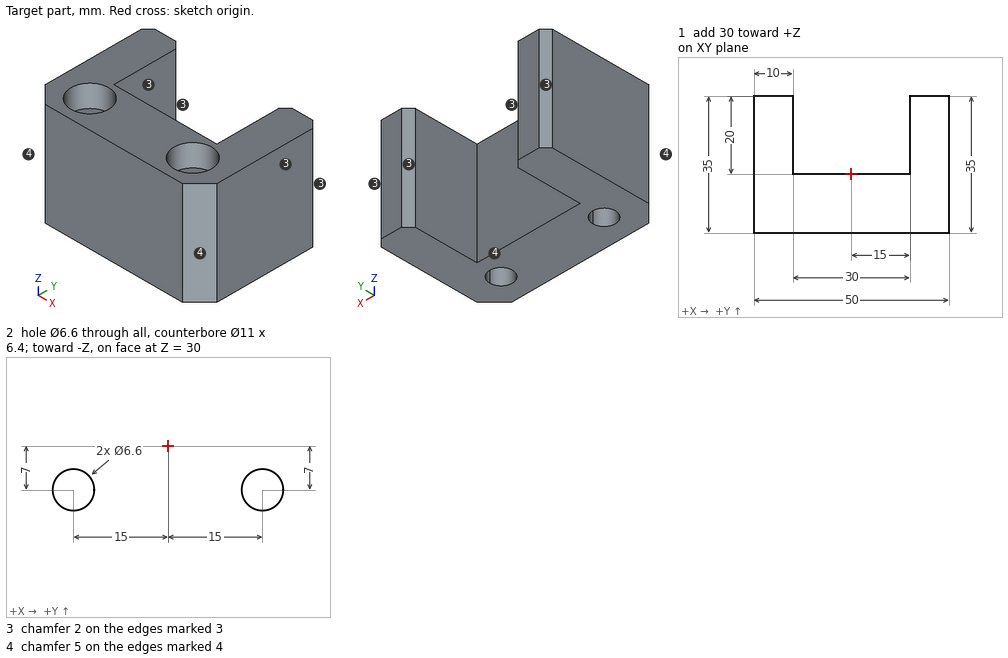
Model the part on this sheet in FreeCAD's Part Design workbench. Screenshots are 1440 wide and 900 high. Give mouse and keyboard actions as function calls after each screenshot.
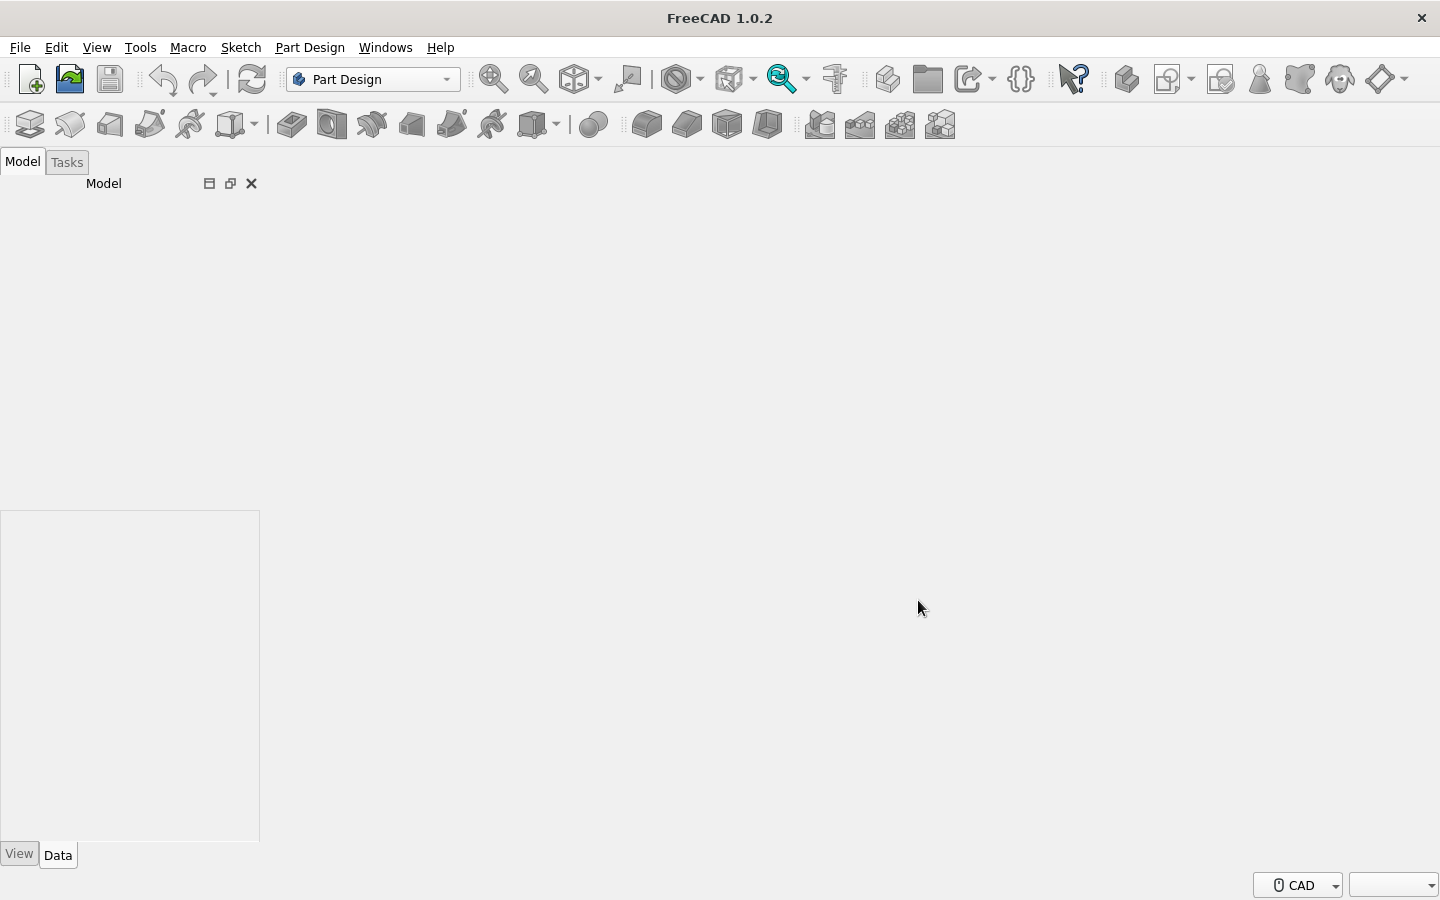
click(30, 80)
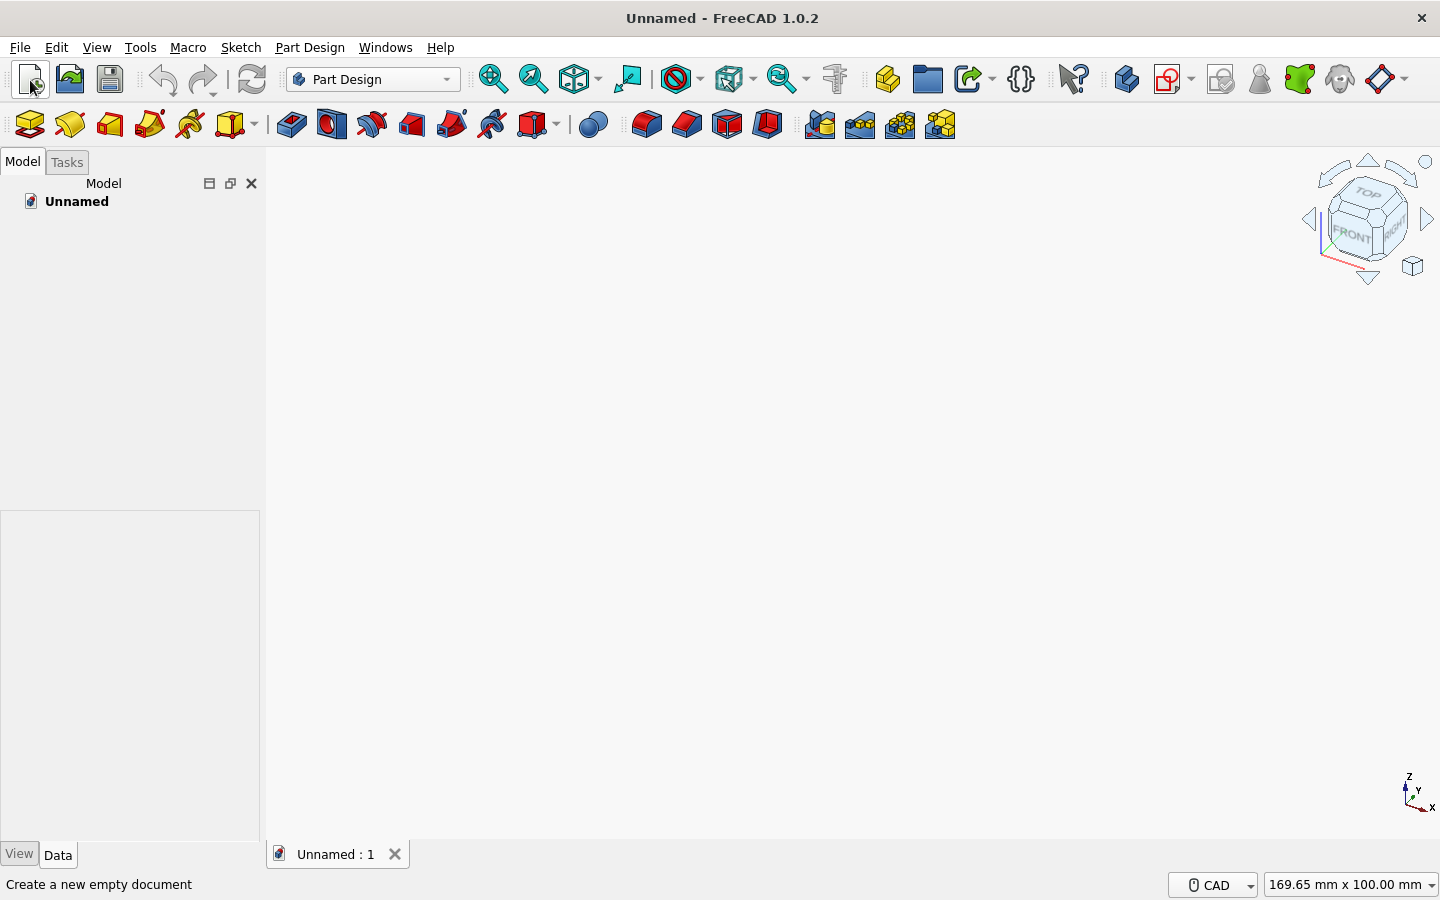
click(1168, 80)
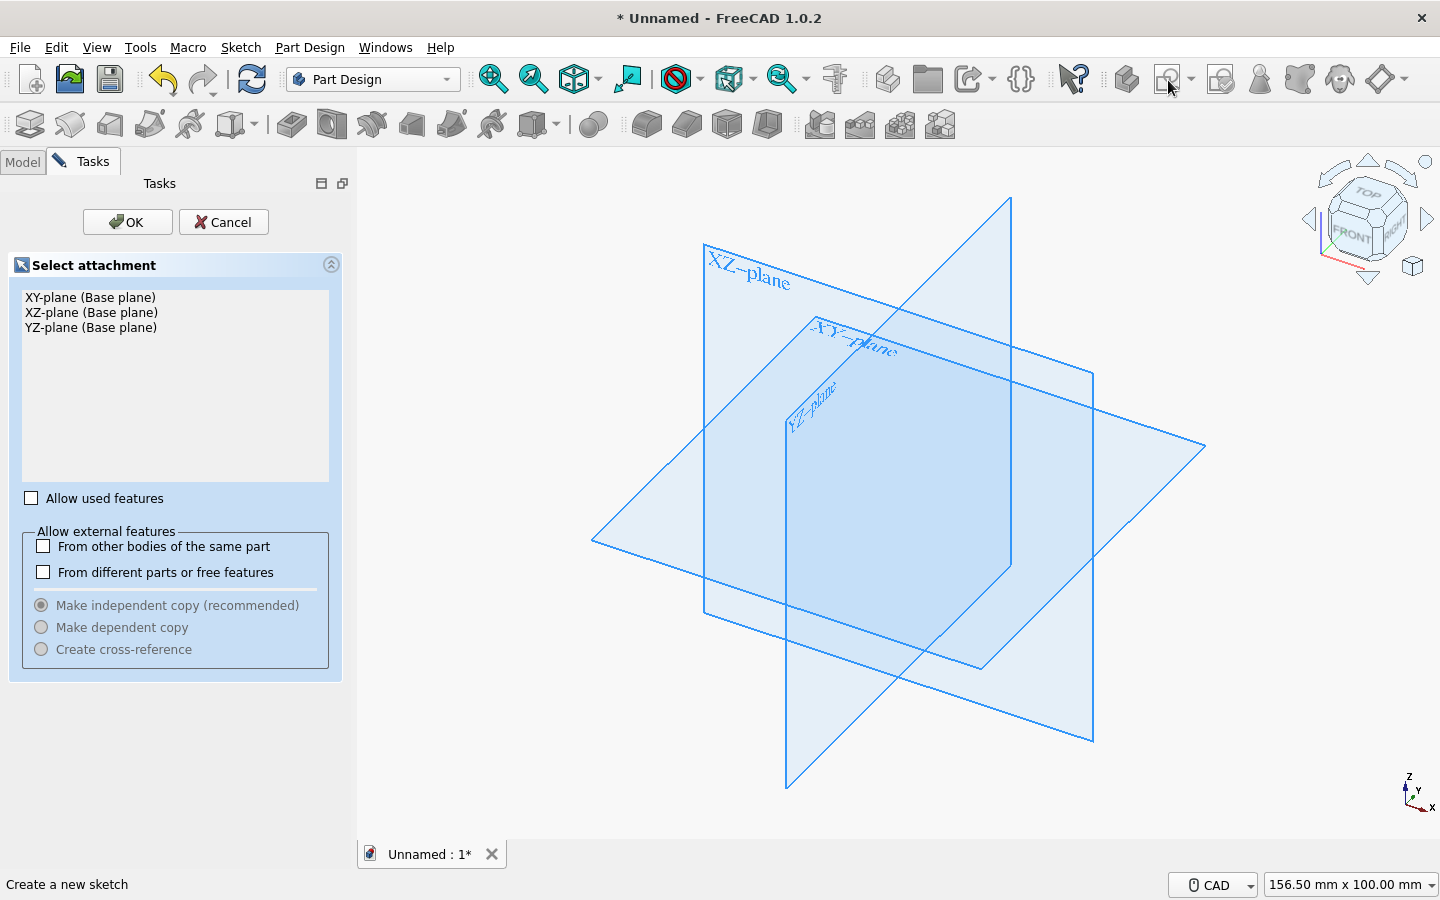
click(82, 298)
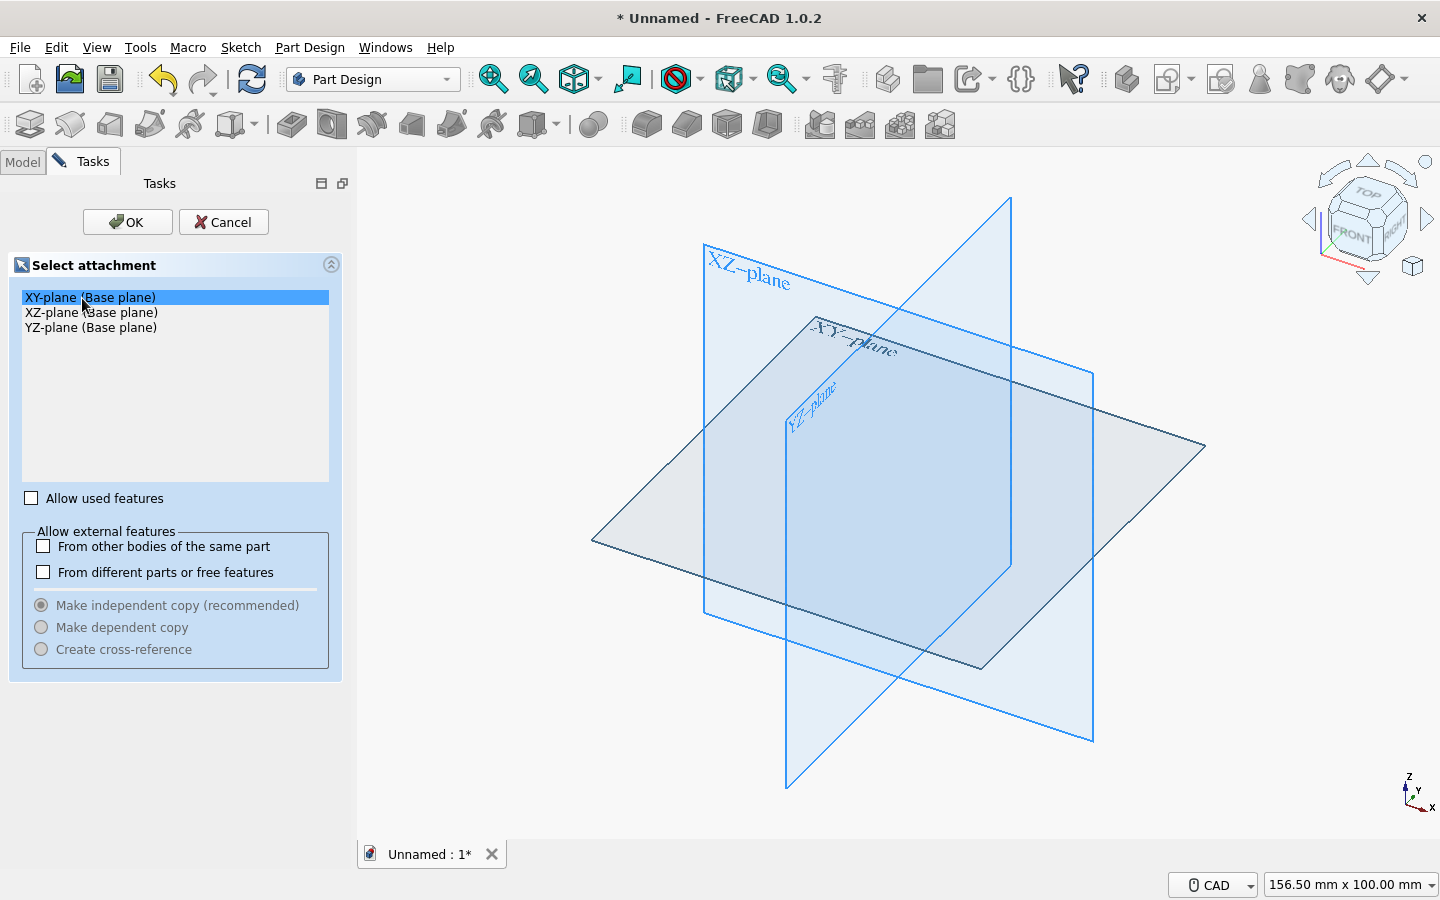
click(128, 222)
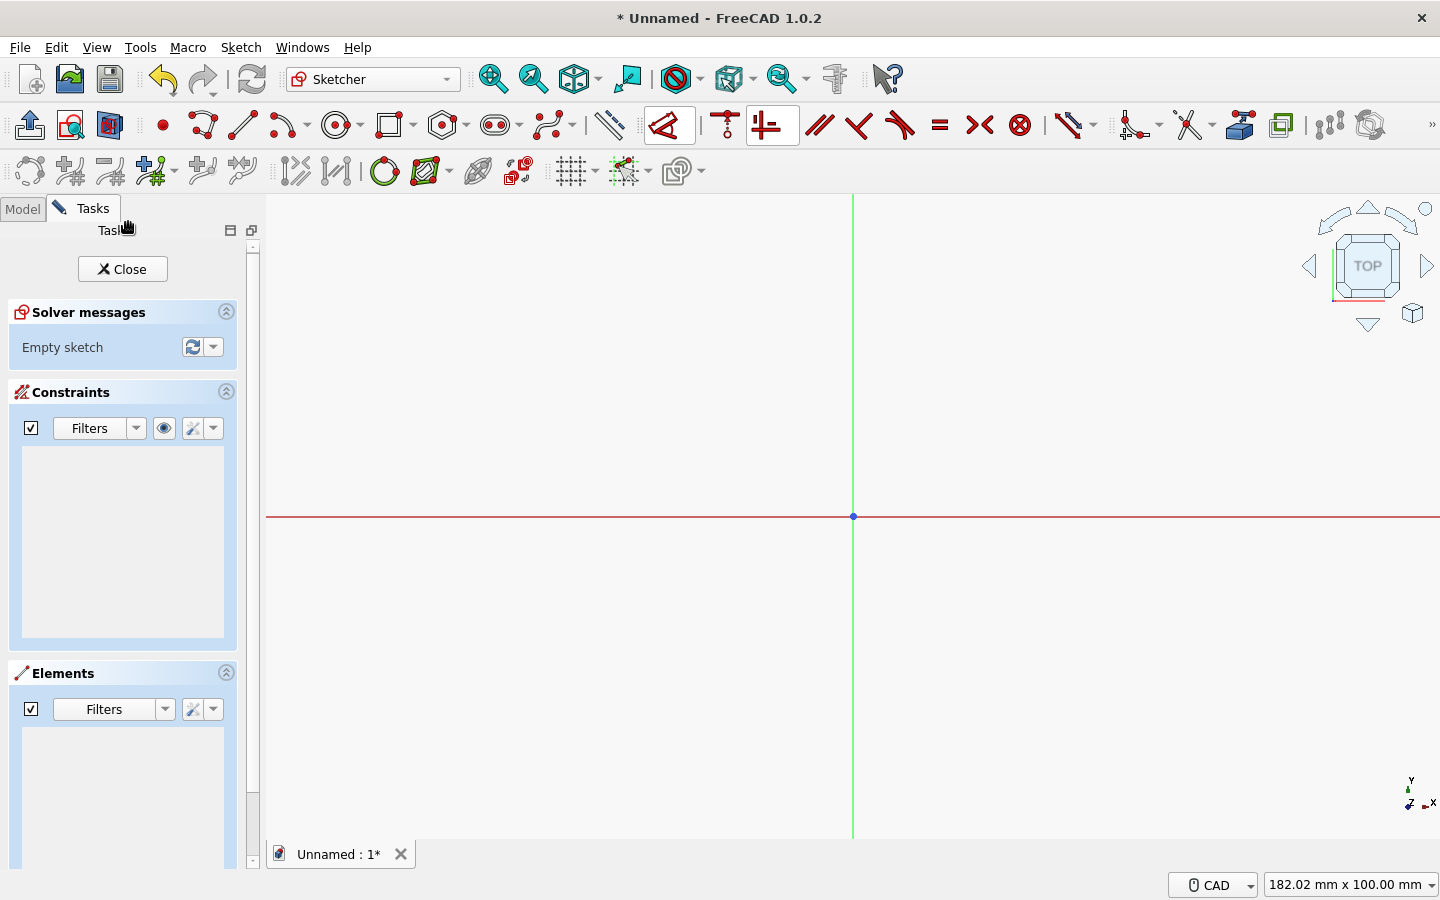
scroll(936, 481, up, 3)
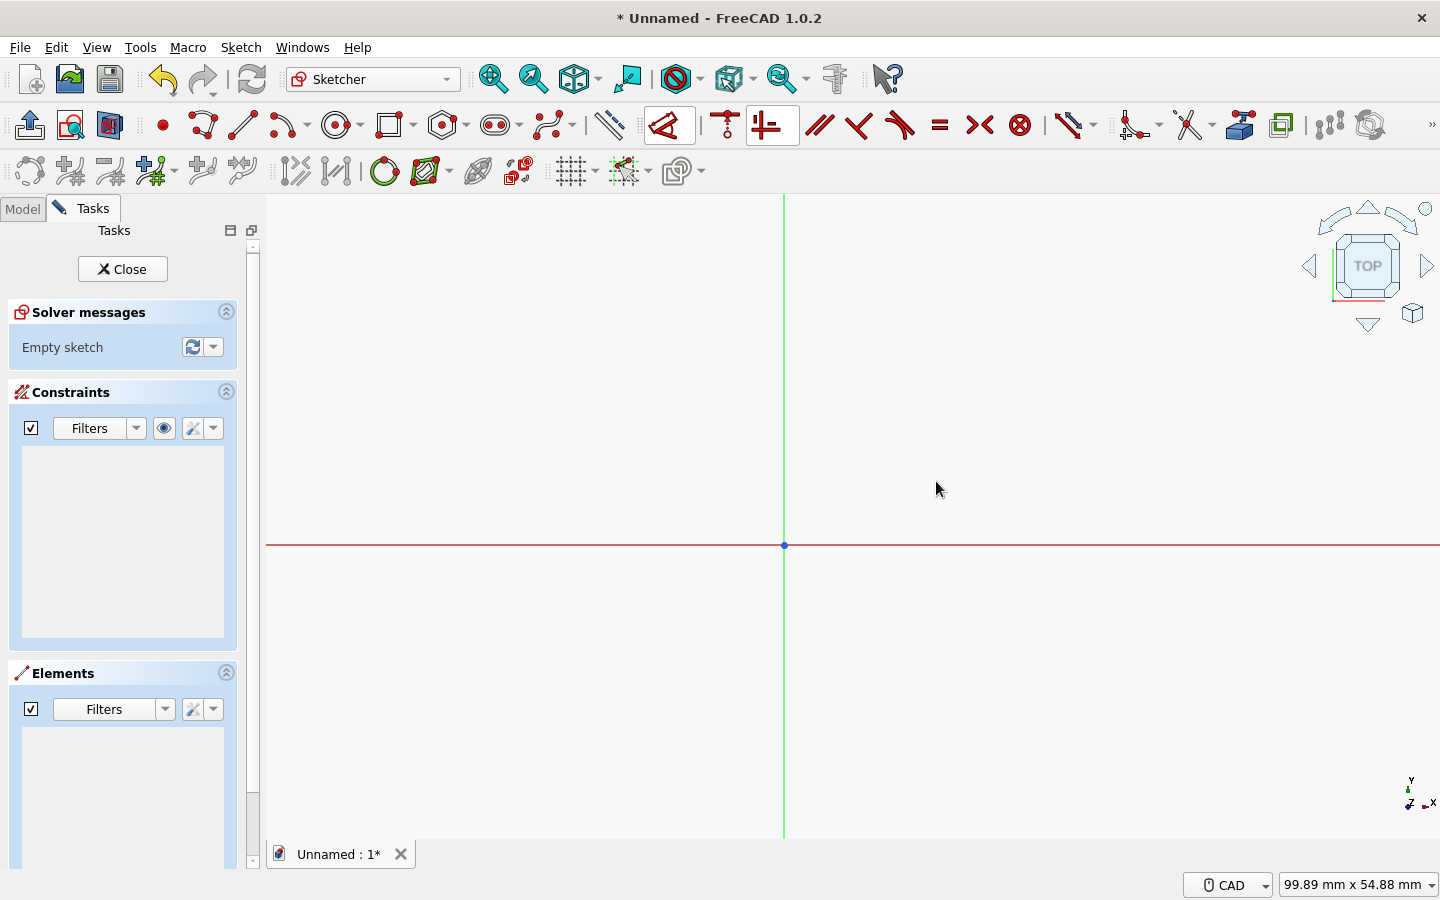
click(204, 126)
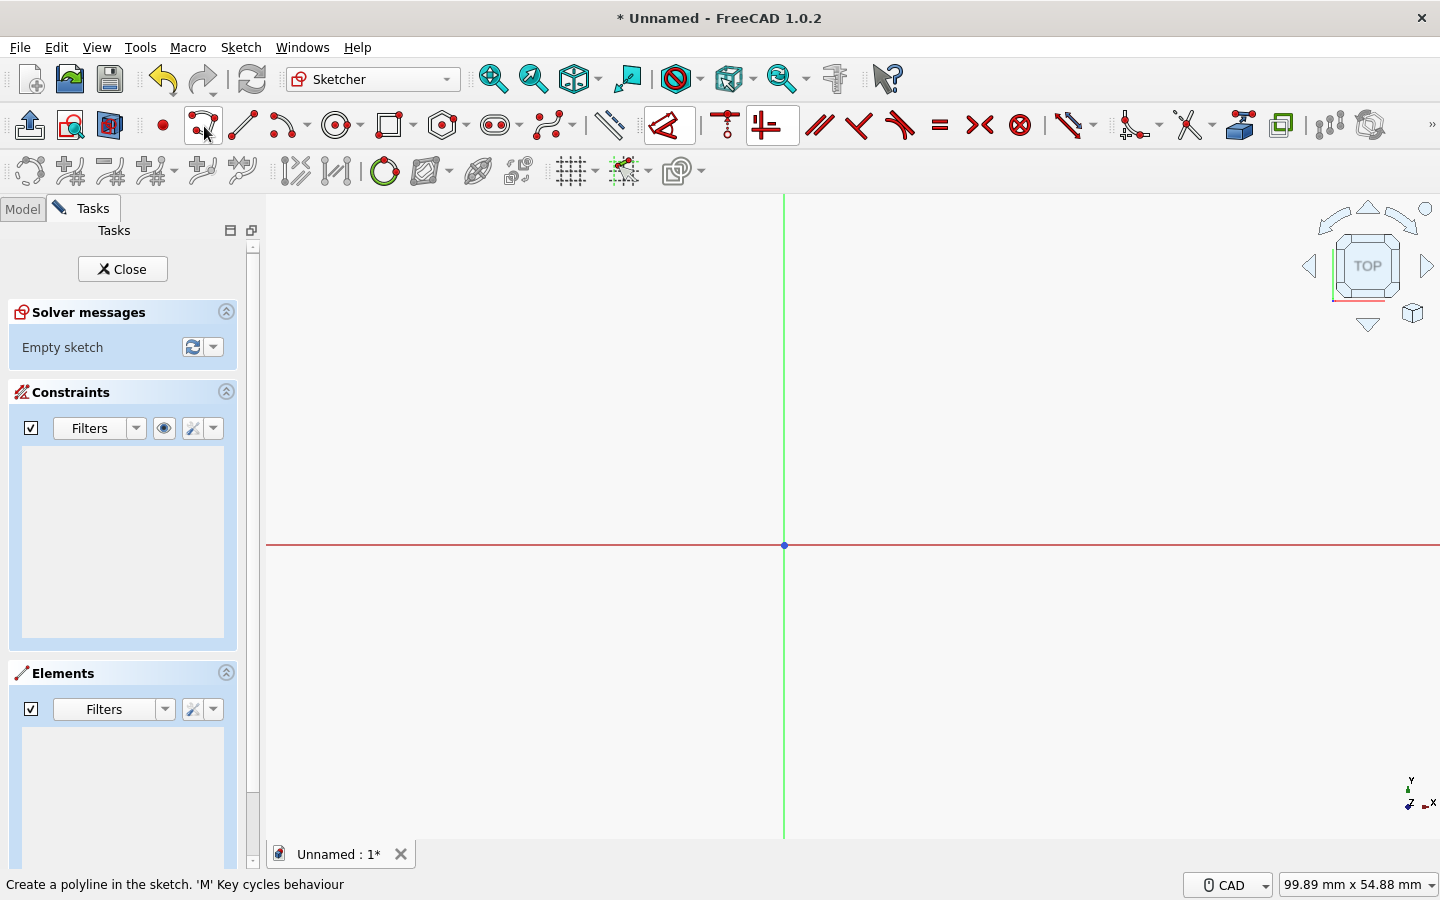
click(961, 545)
click(608, 536)
click(608, 310)
click(490, 310)
click(490, 722)
click(1078, 722)
click(1078, 310)
click(961, 310)
click(961, 545)
key(Escape)
key(Escape)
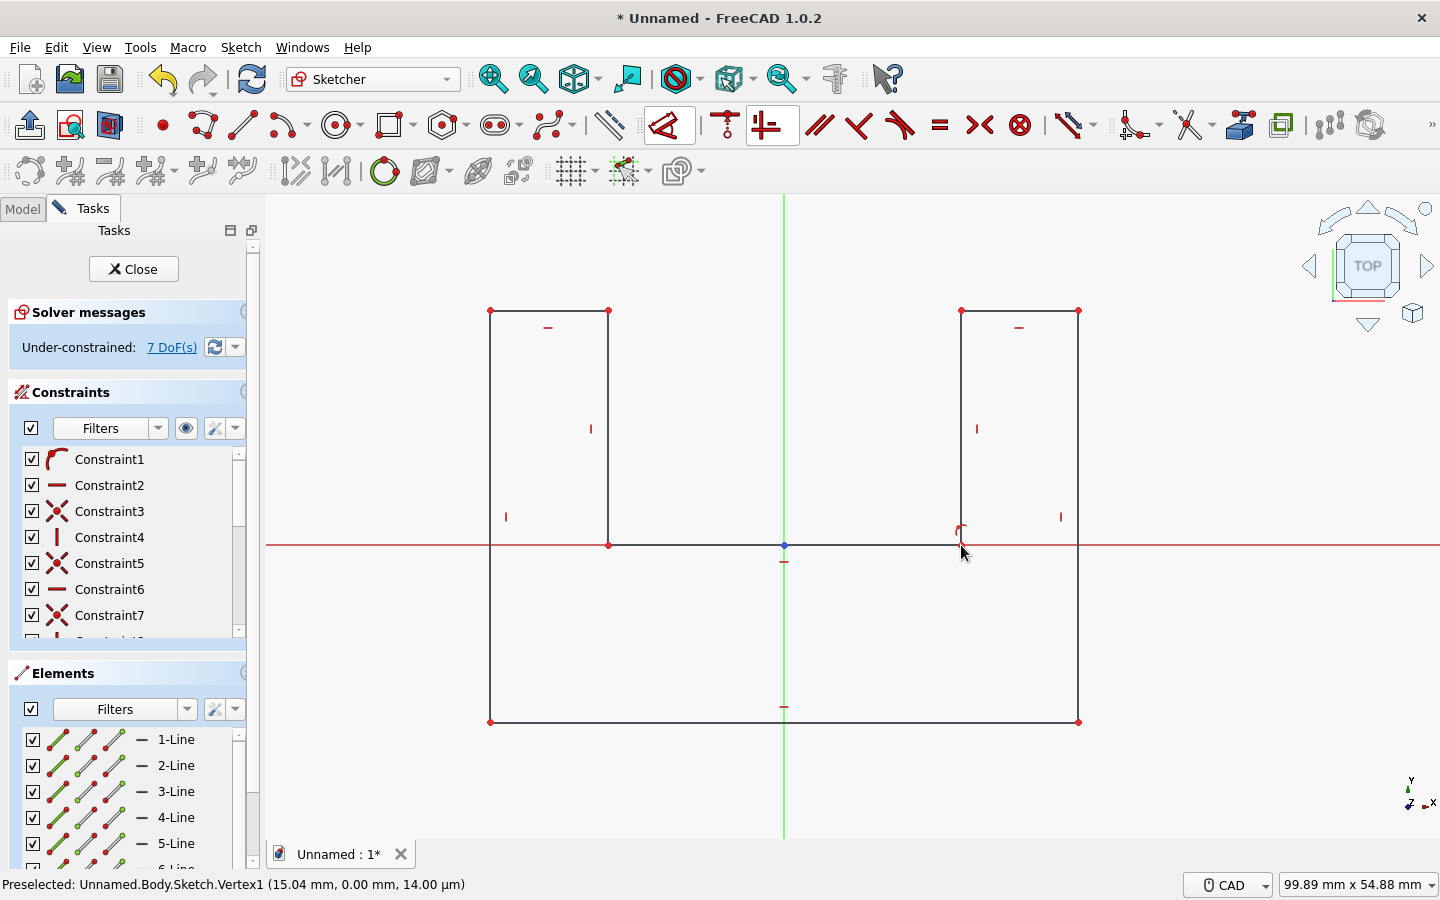
click(664, 126)